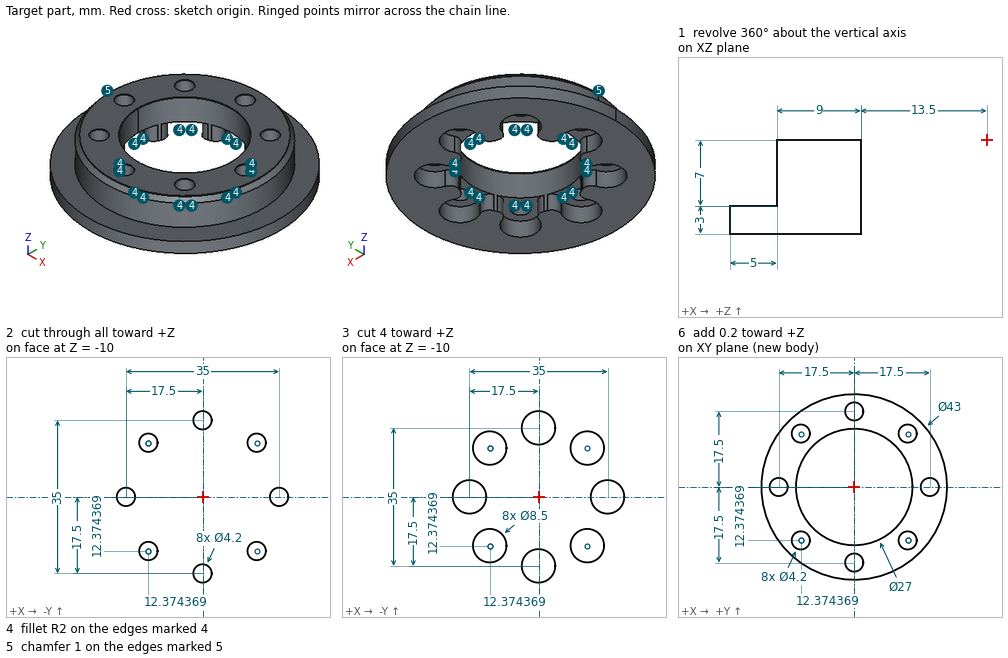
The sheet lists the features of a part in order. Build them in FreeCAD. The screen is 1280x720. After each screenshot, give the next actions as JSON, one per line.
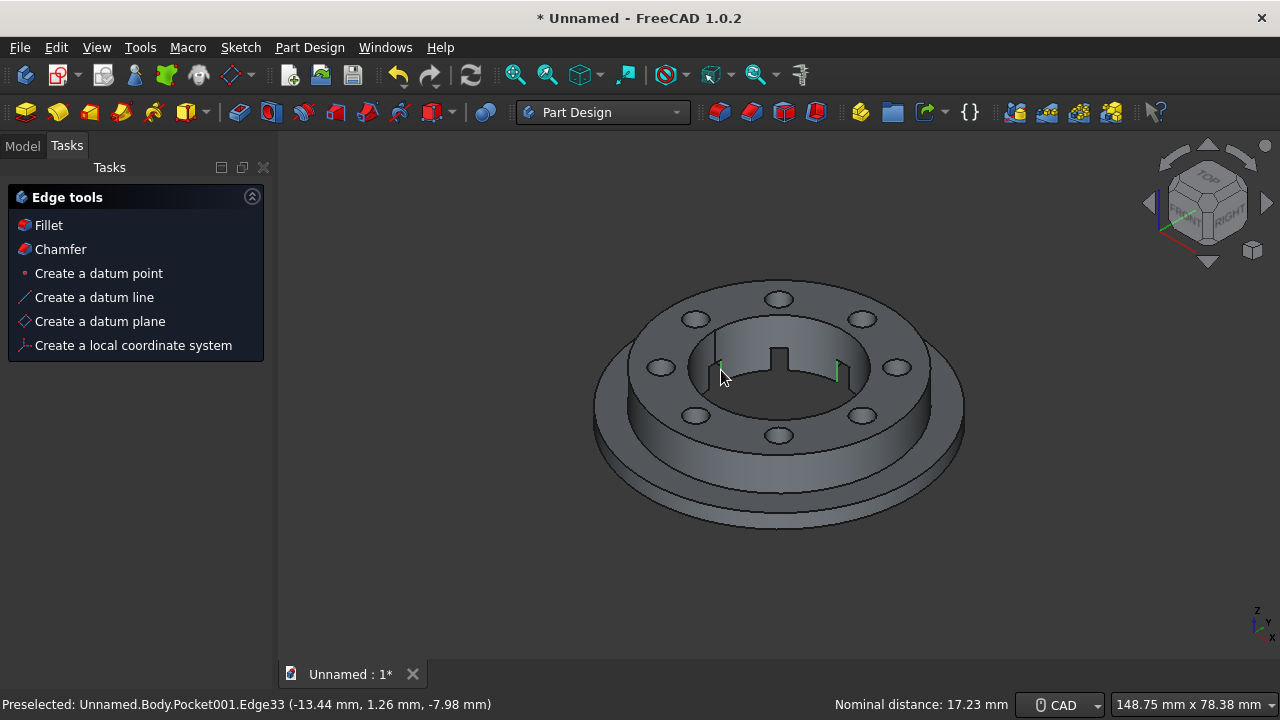
{"action": "key", "text": "2"}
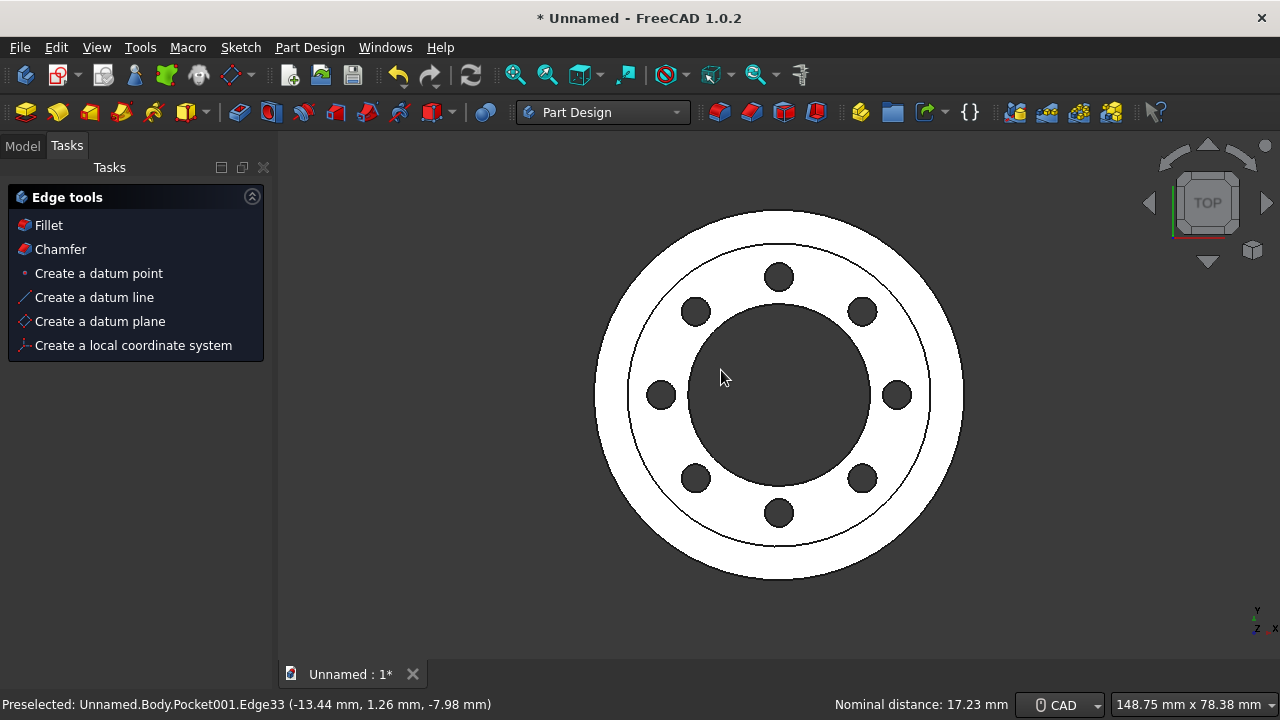
{"action": "key", "text": "1"}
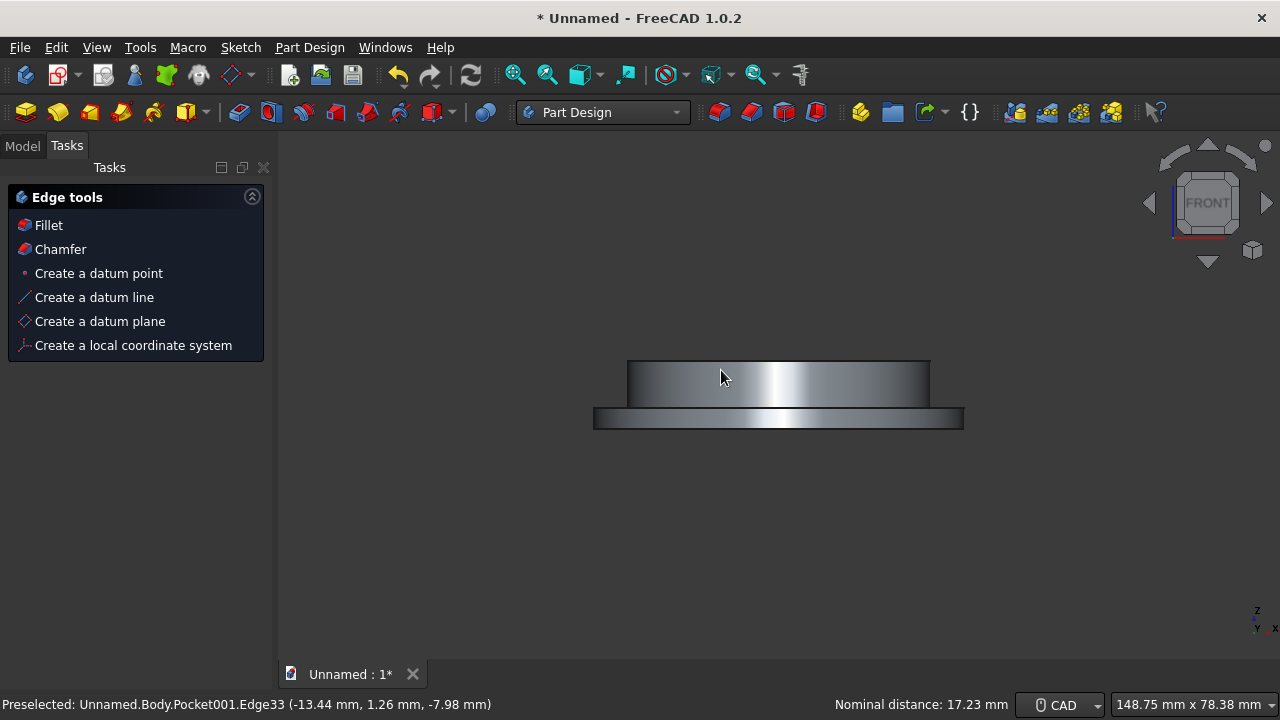
{"action": "left_click", "coordinate": [516, 76]}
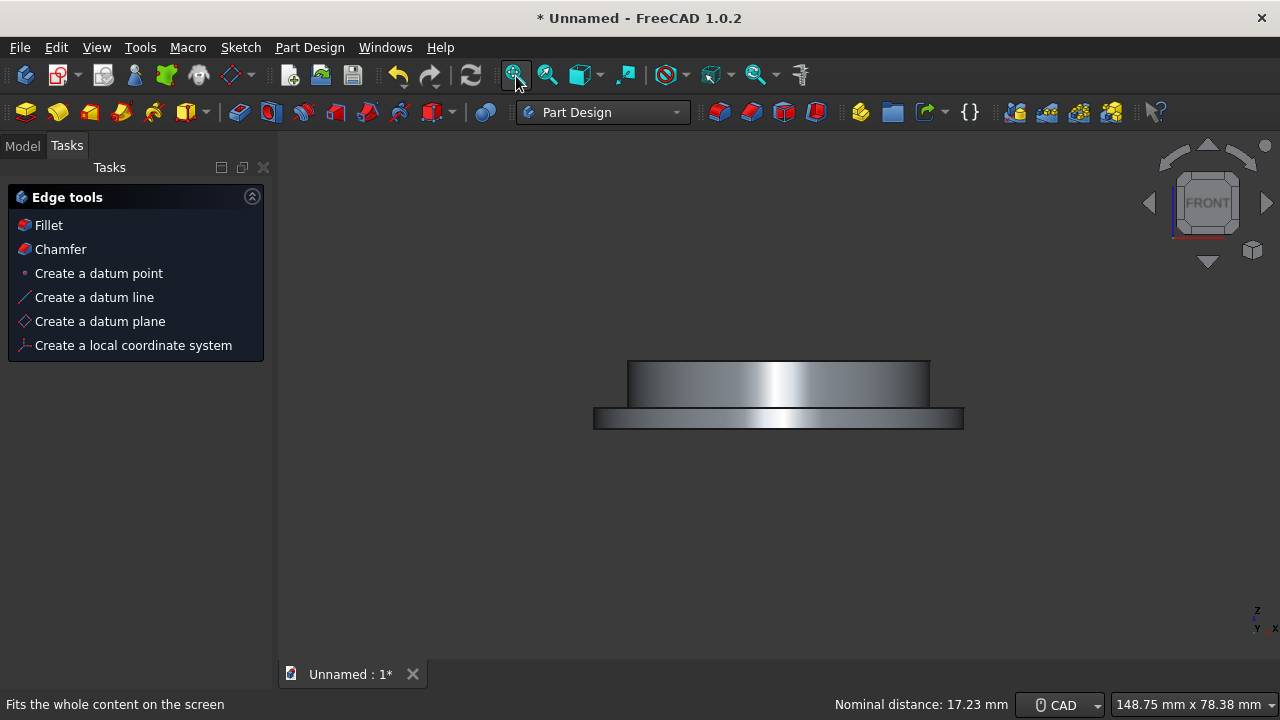
{"action": "key", "text": "3"}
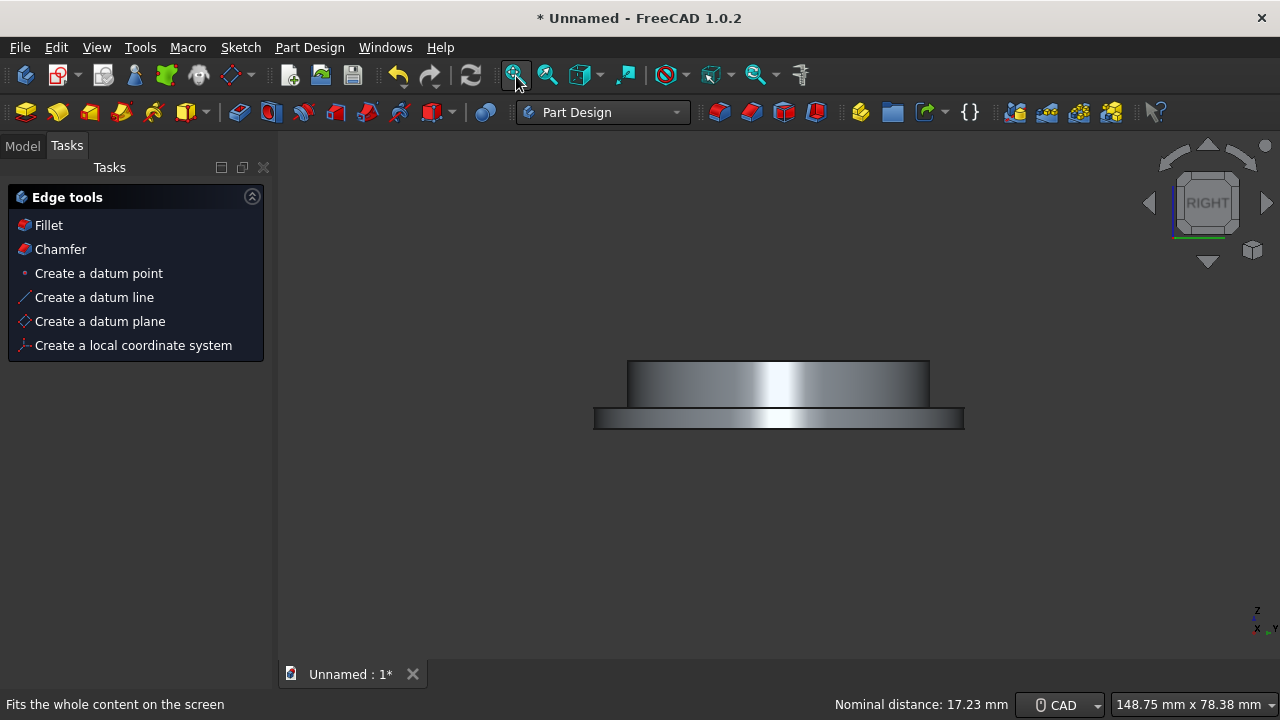
{"action": "left_click", "coordinate": [516, 76]}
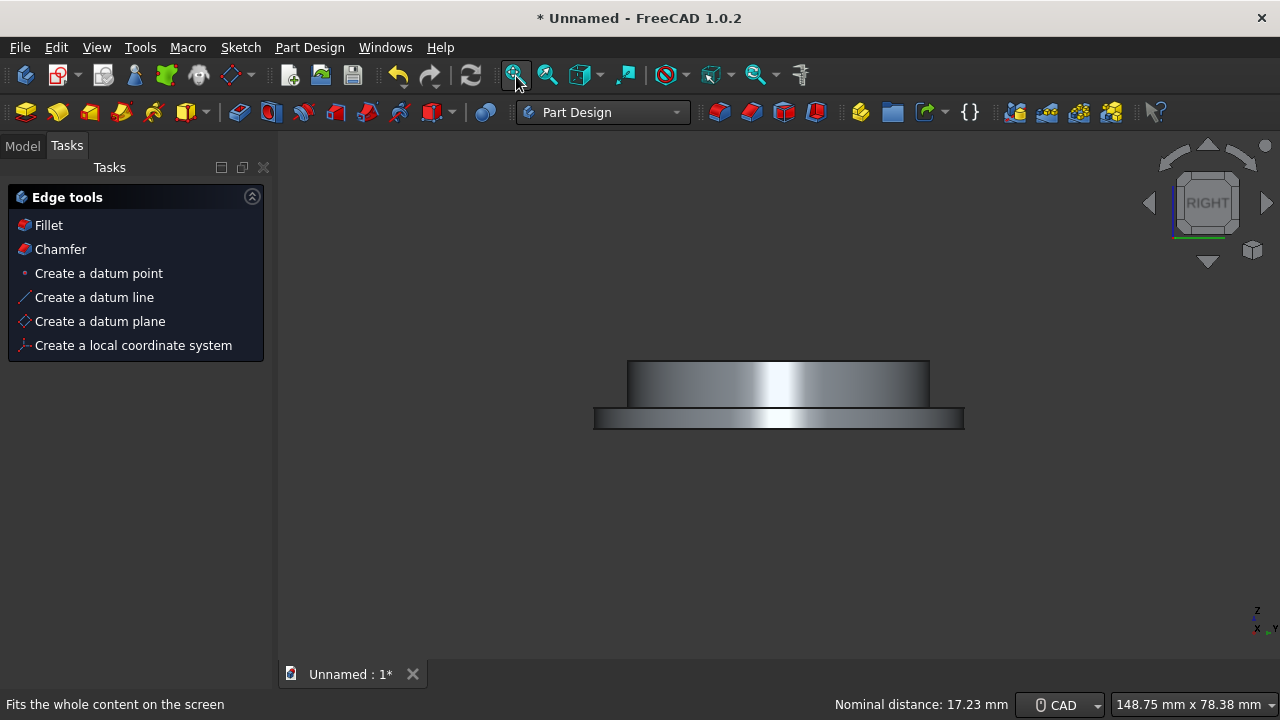
{"action": "key", "text": "5"}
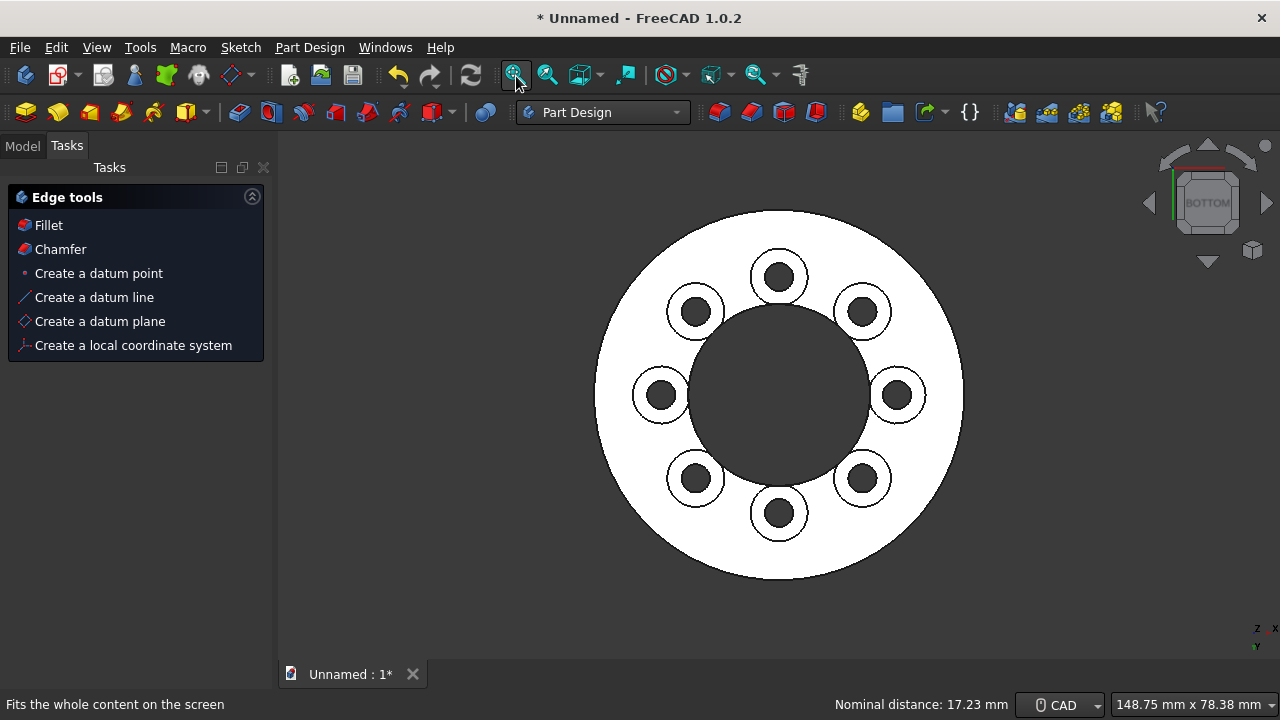
{"action": "key", "text": "4"}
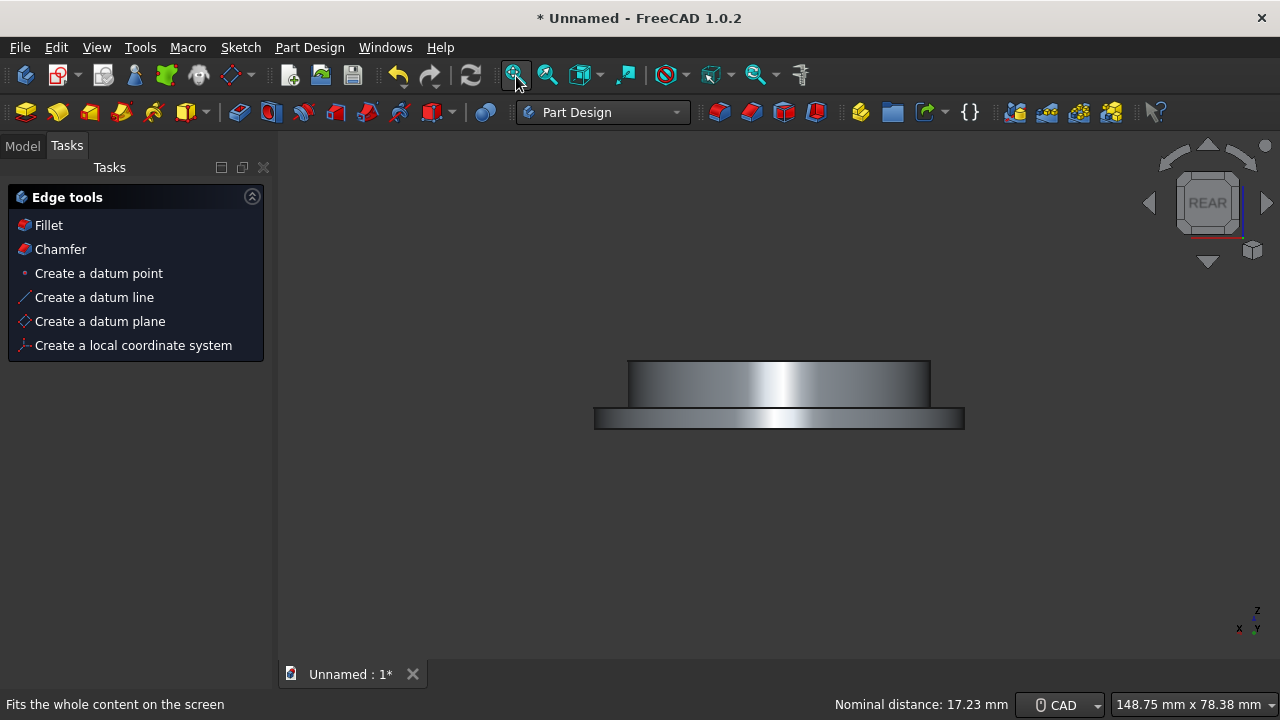
{"action": "left_click", "coordinate": [516, 76]}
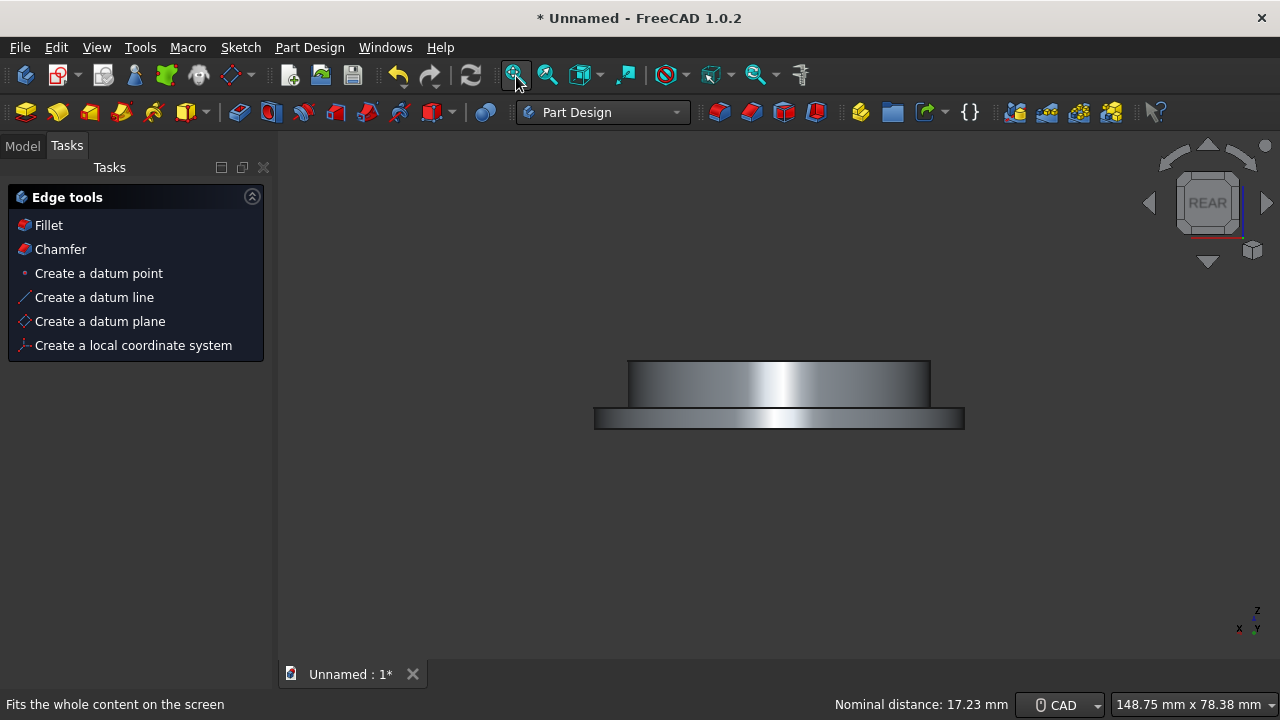
{"action": "key", "text": "6"}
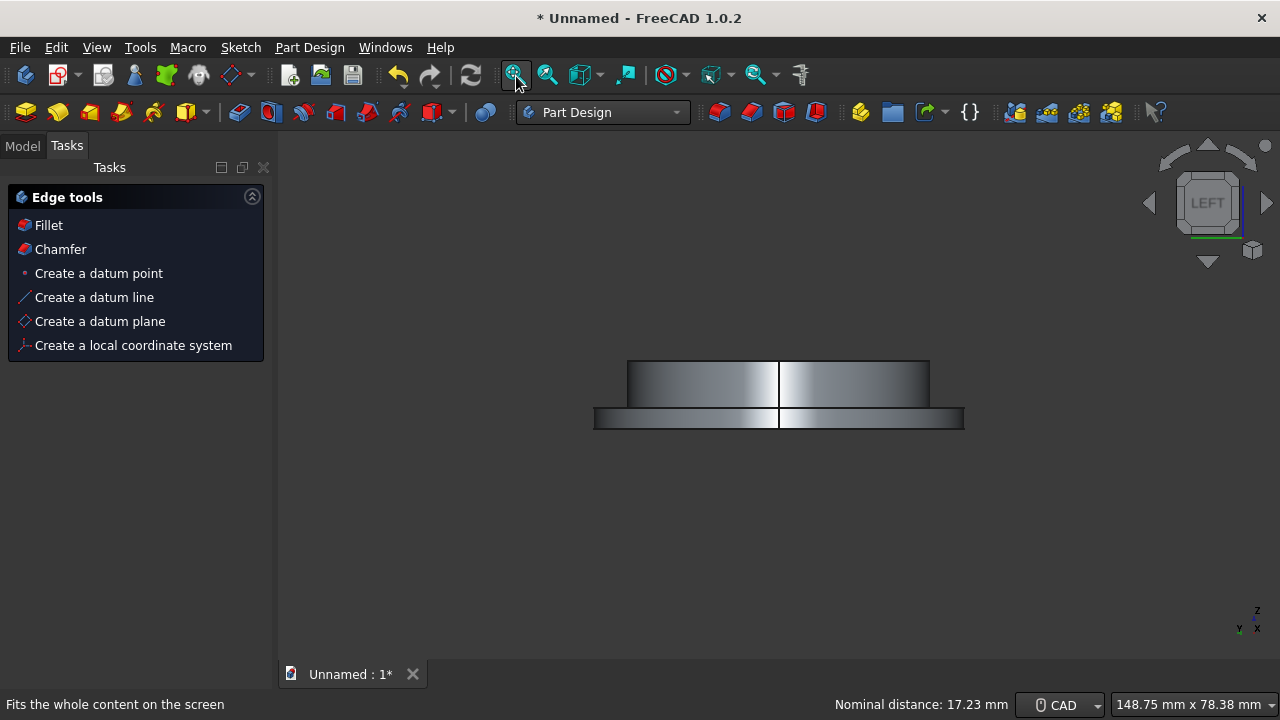
{"action": "key", "text": "v f"}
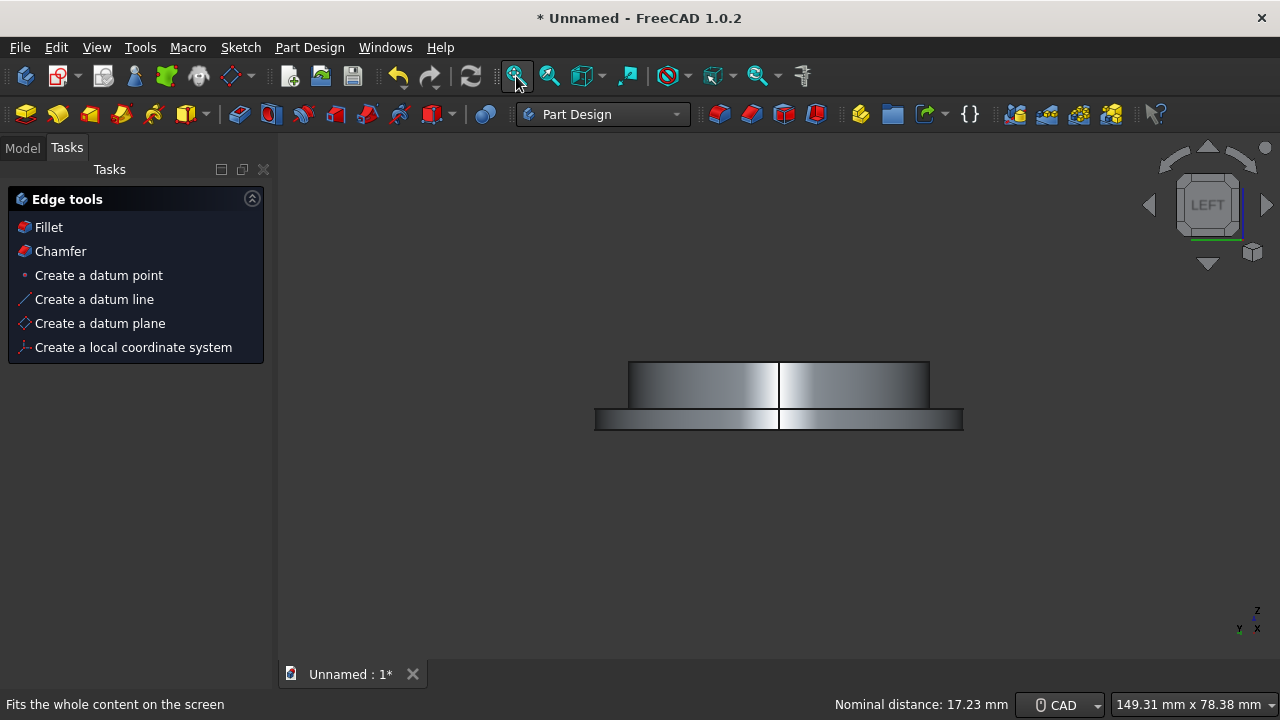
{"action": "key", "text": "v 3"}